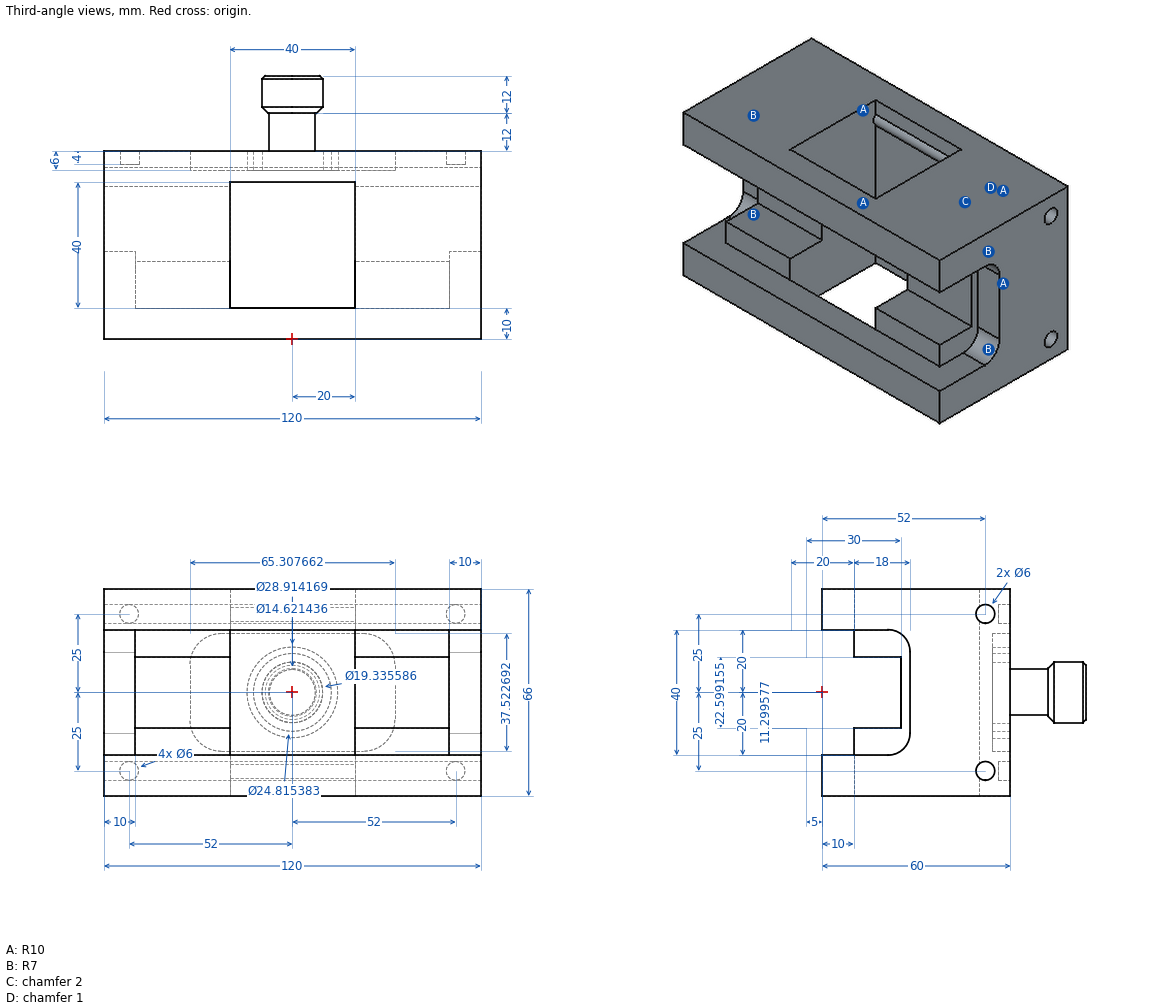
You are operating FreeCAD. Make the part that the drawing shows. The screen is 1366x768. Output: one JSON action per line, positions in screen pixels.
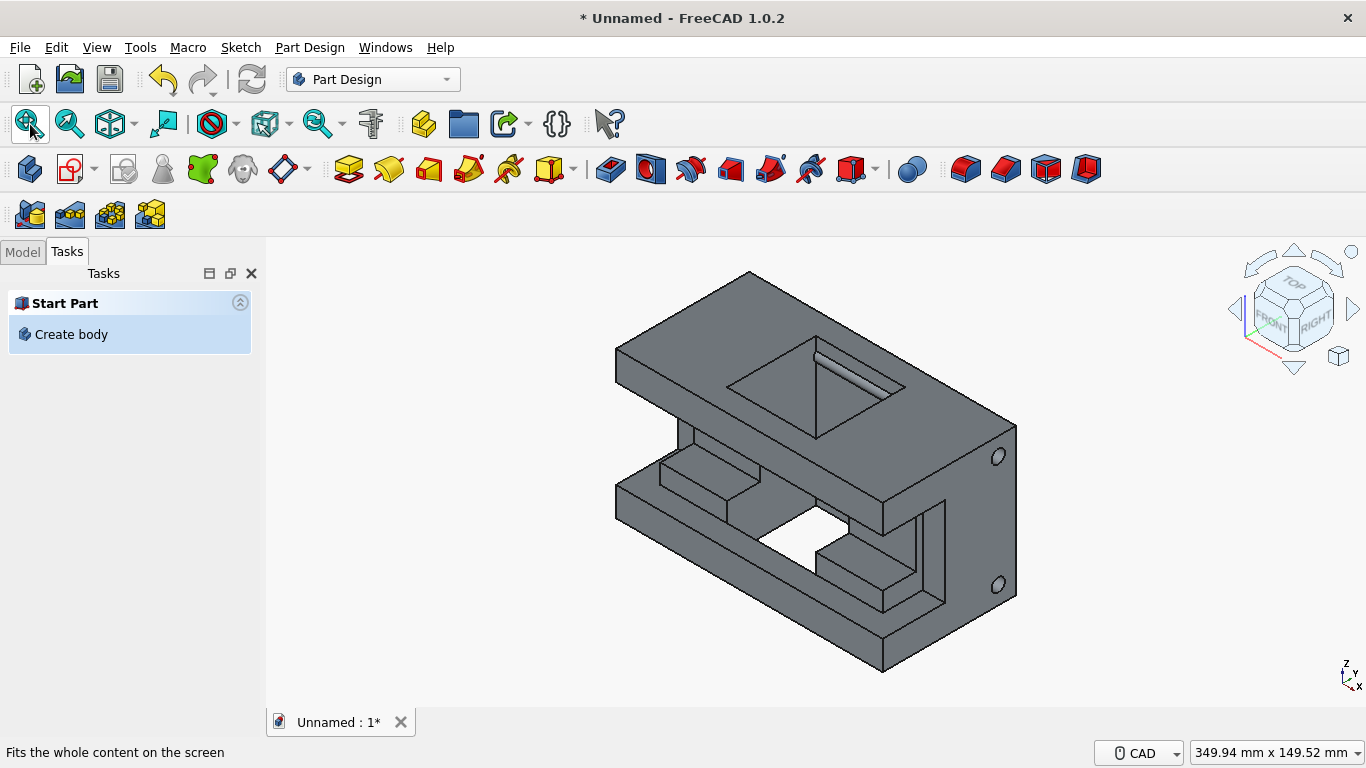
{"action": "key", "text": "2"}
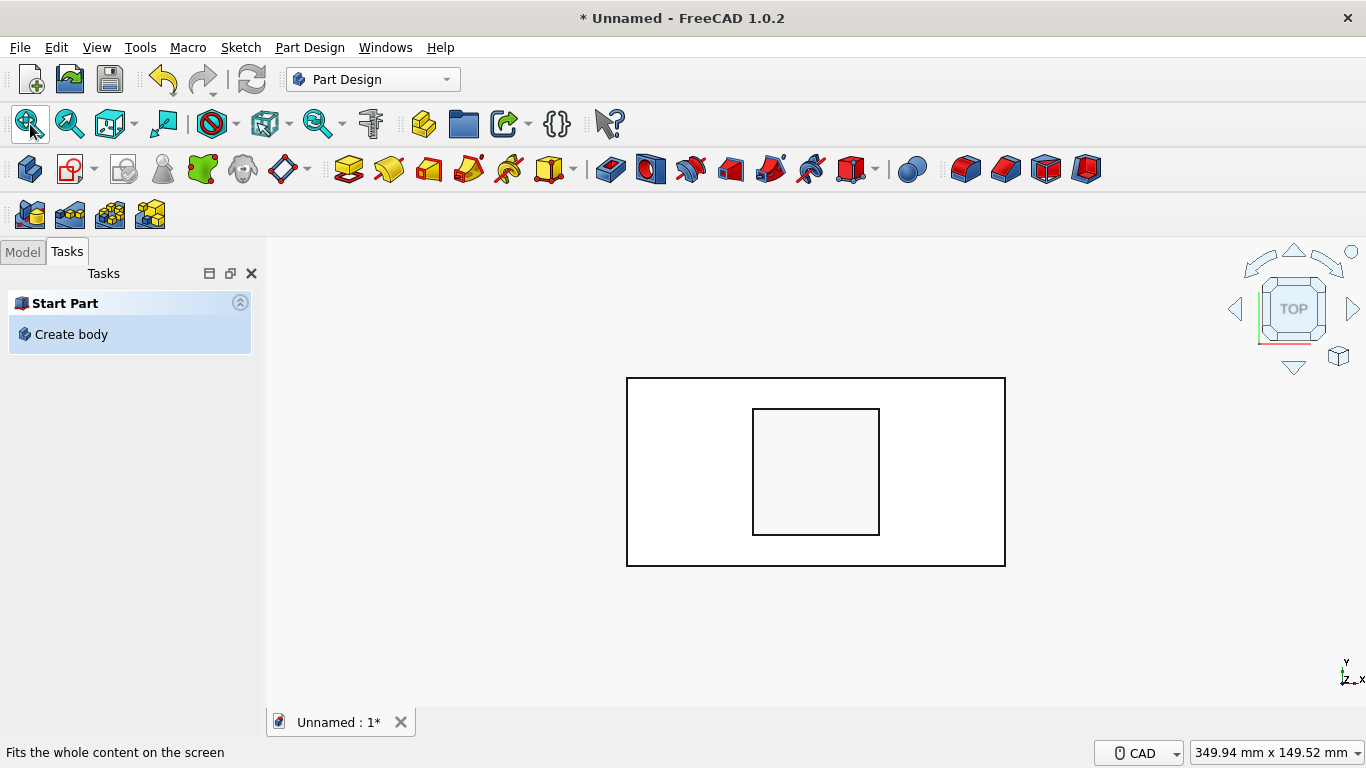
{"action": "left_click", "coordinate": [30, 124]}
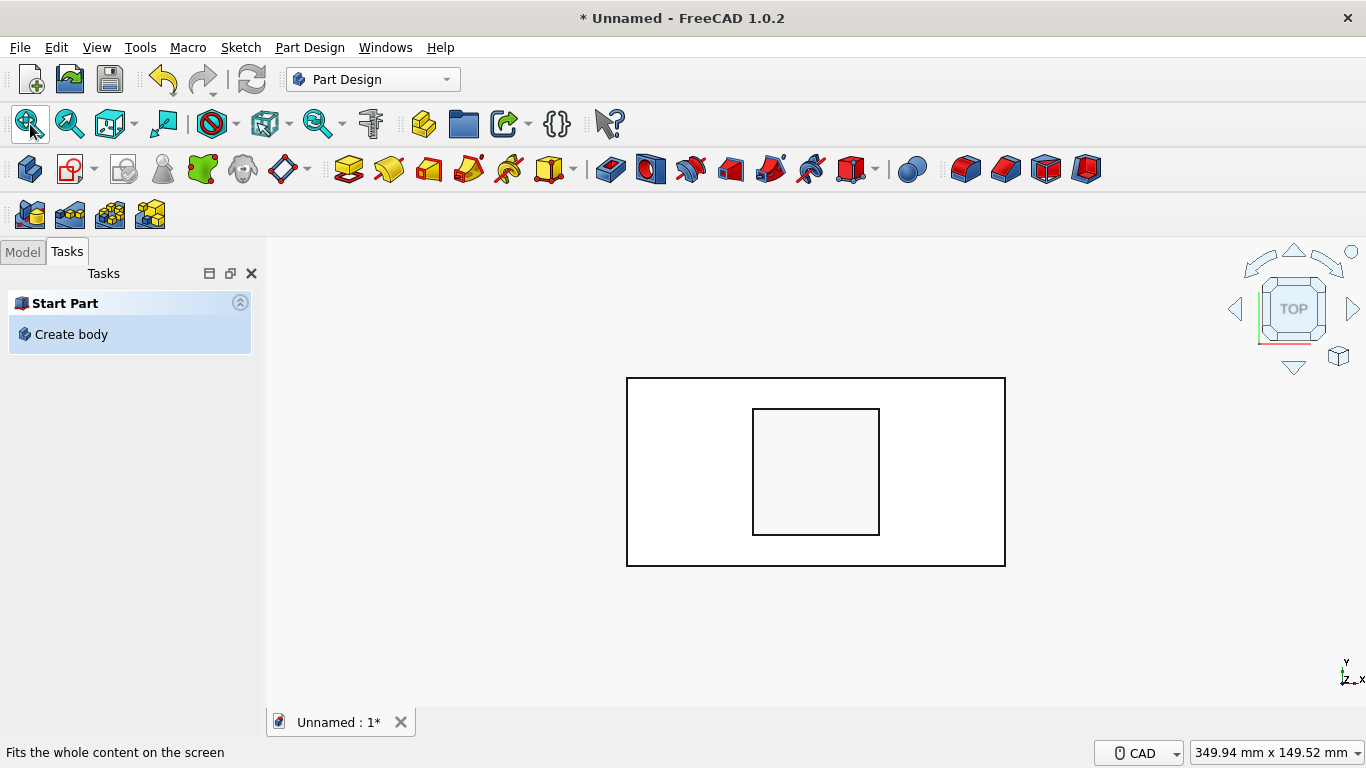
{"action": "key", "text": "1"}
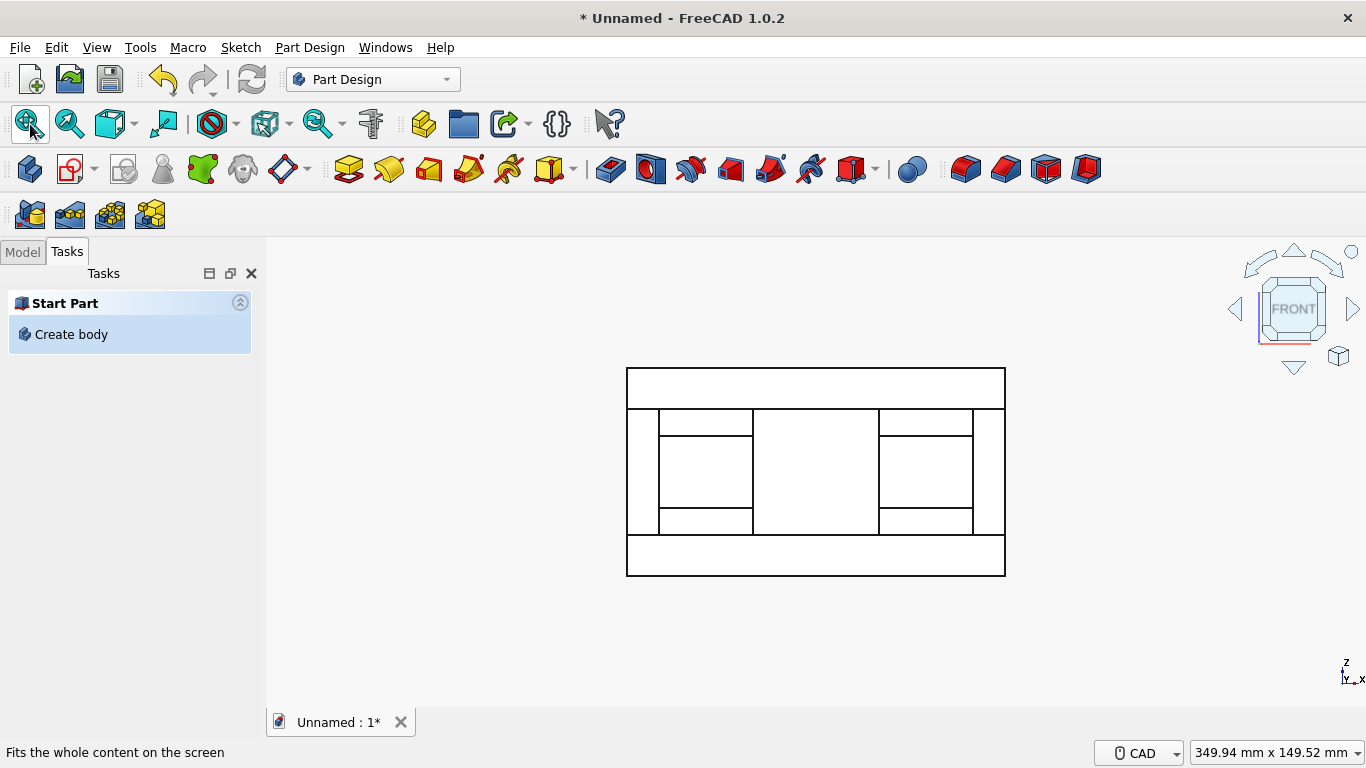
{"action": "left_click", "coordinate": [30, 124]}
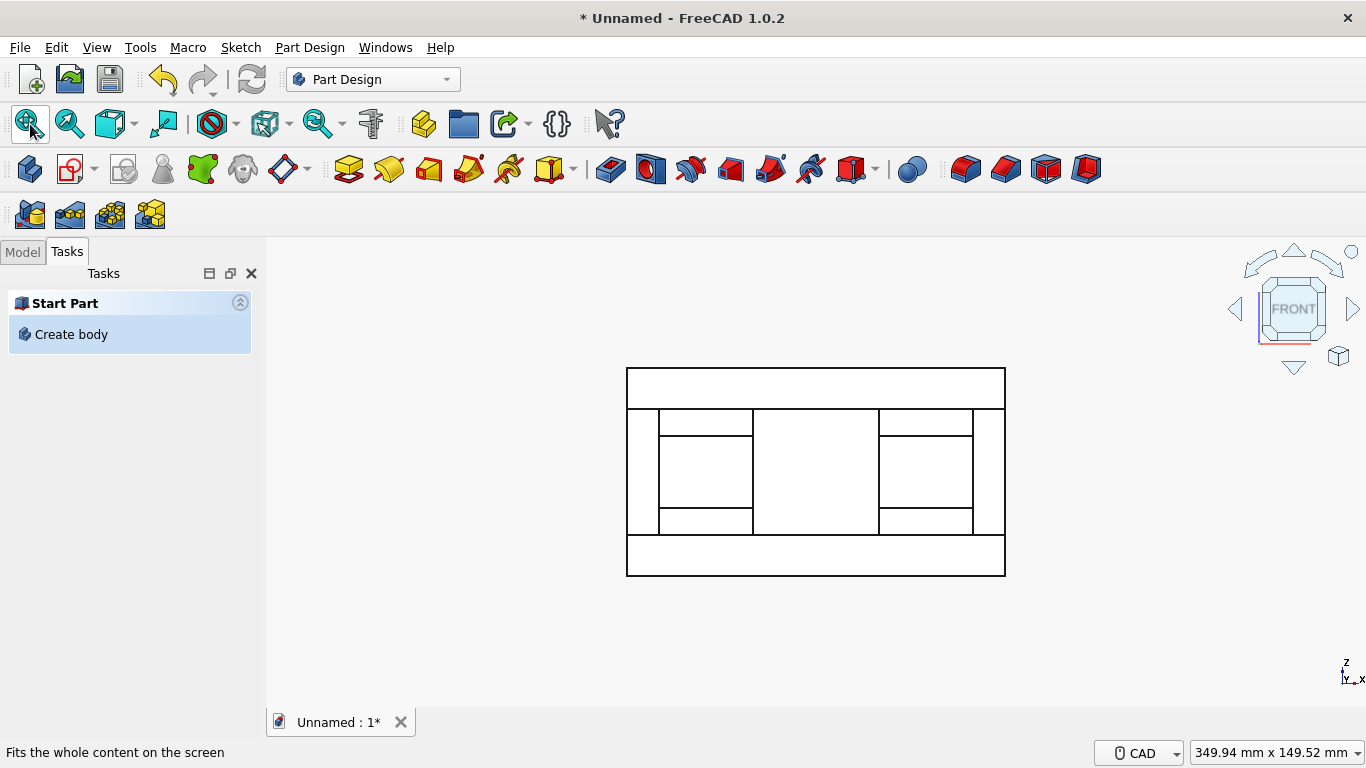
{"action": "key", "text": "3"}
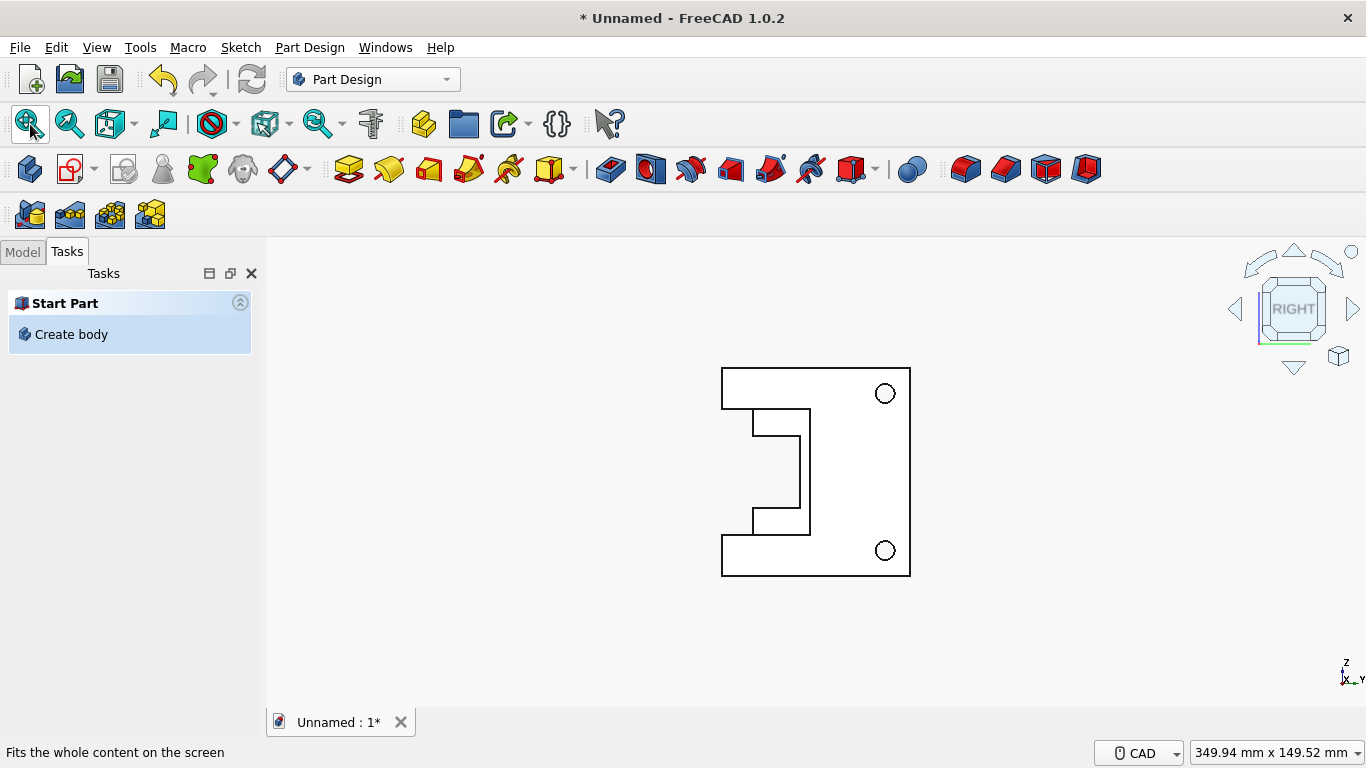
{"action": "left_click", "coordinate": [30, 124]}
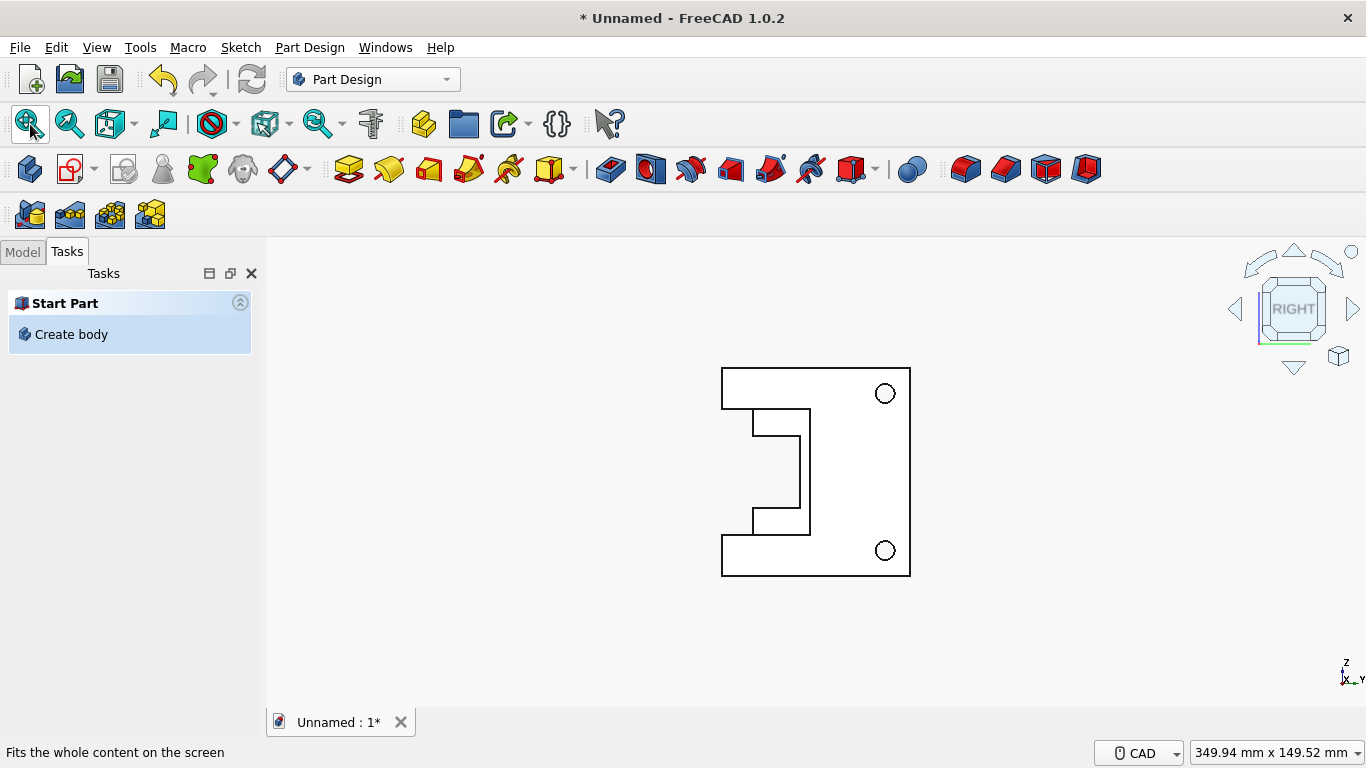
{"action": "key", "text": "5"}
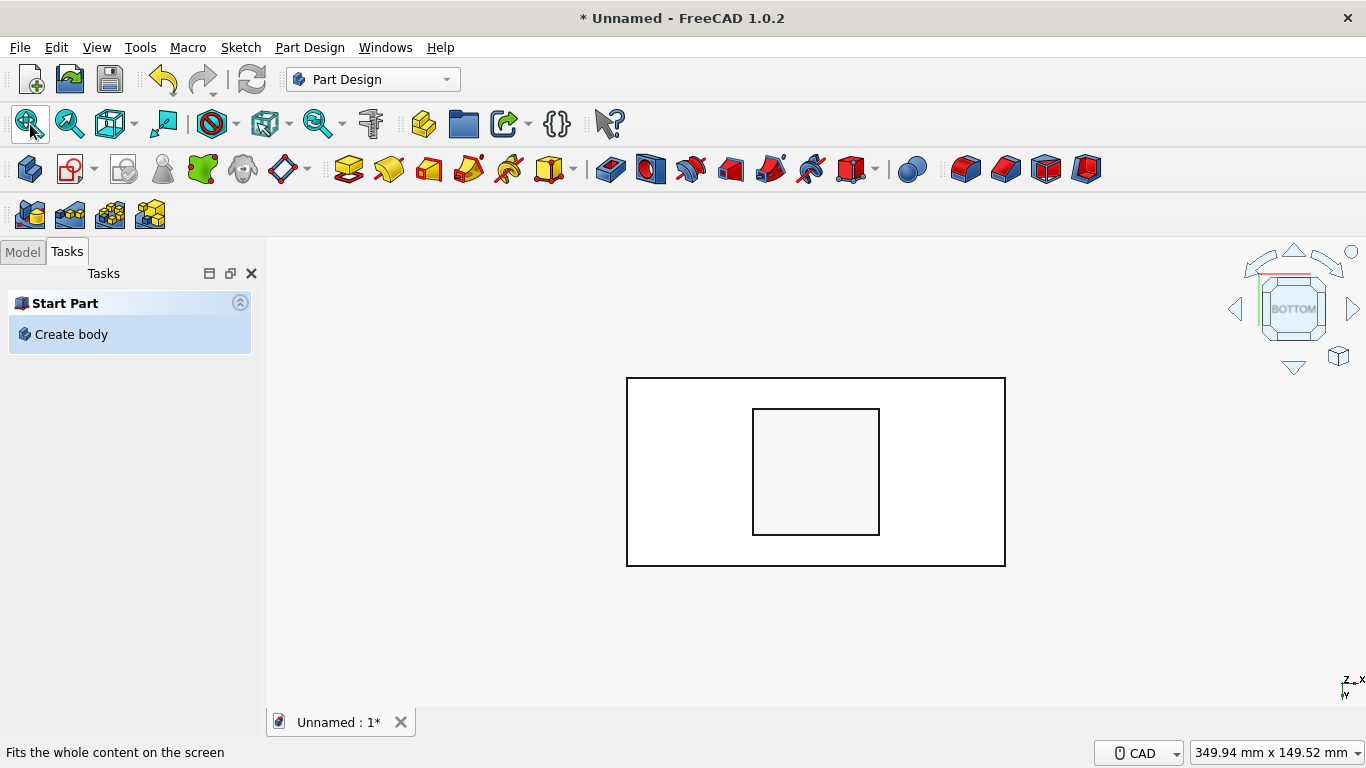
{"action": "left_click", "coordinate": [30, 124]}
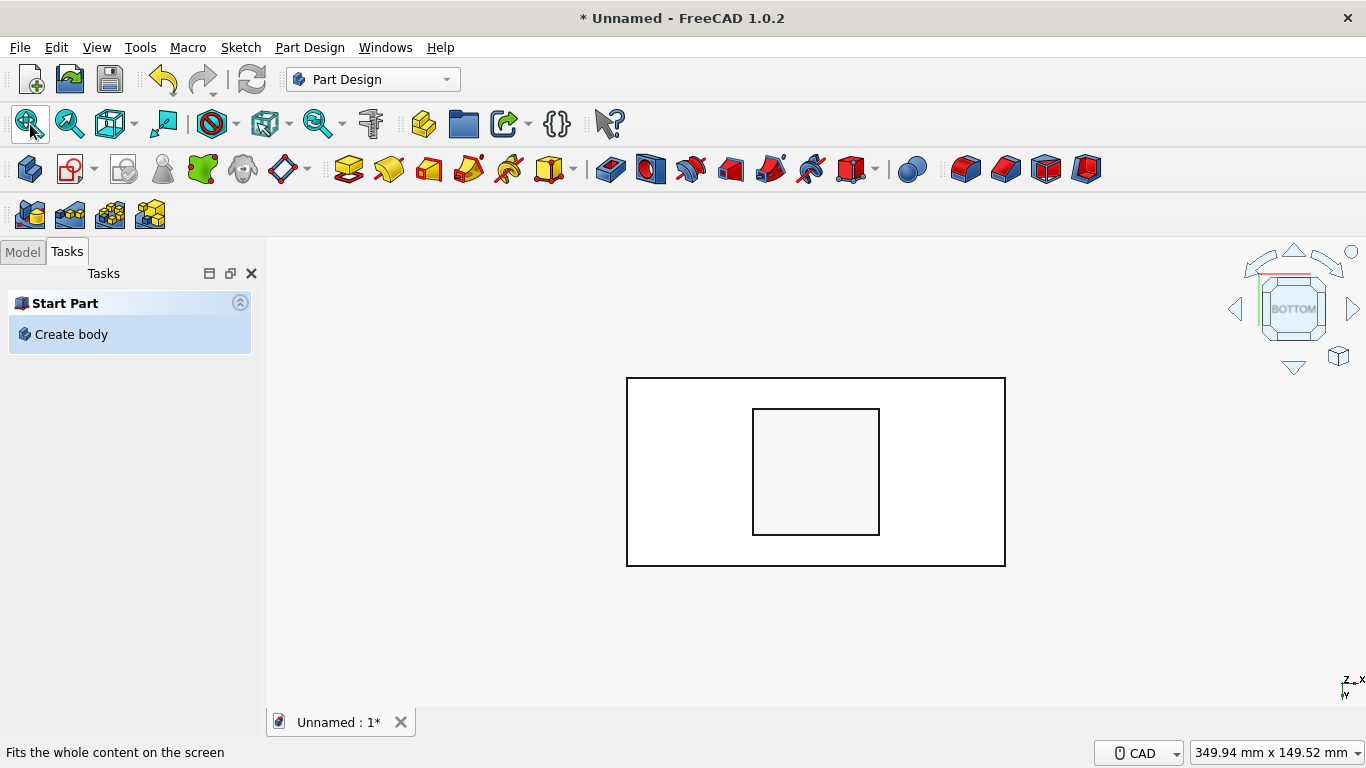
{"action": "key", "text": "4"}